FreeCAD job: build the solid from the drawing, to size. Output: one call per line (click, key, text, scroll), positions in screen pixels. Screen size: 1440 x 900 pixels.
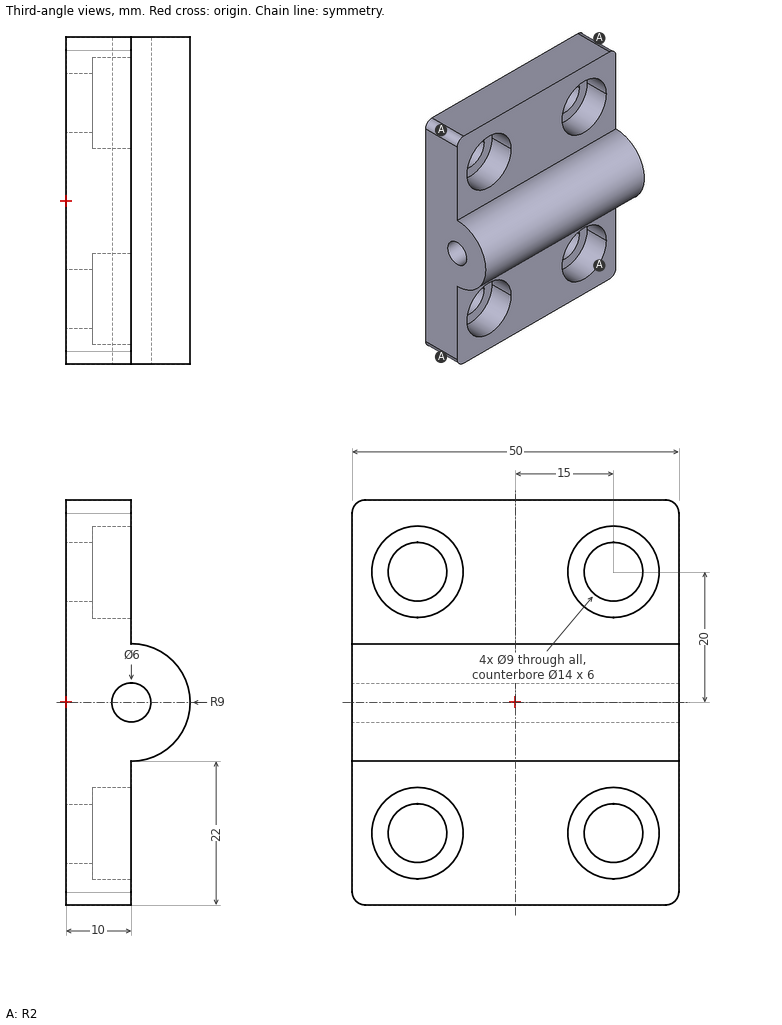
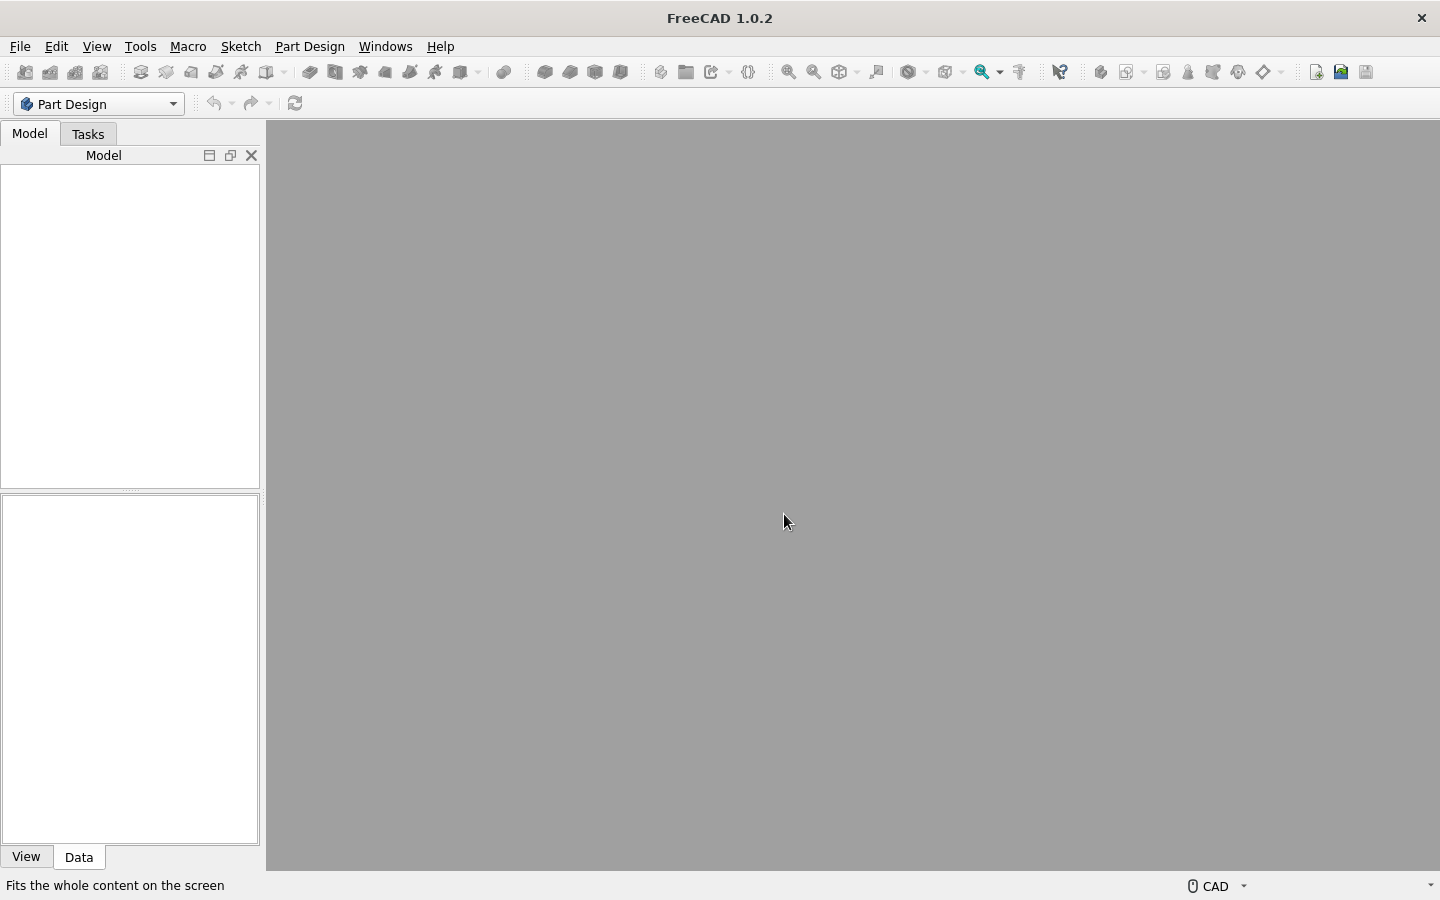
click(1316, 72)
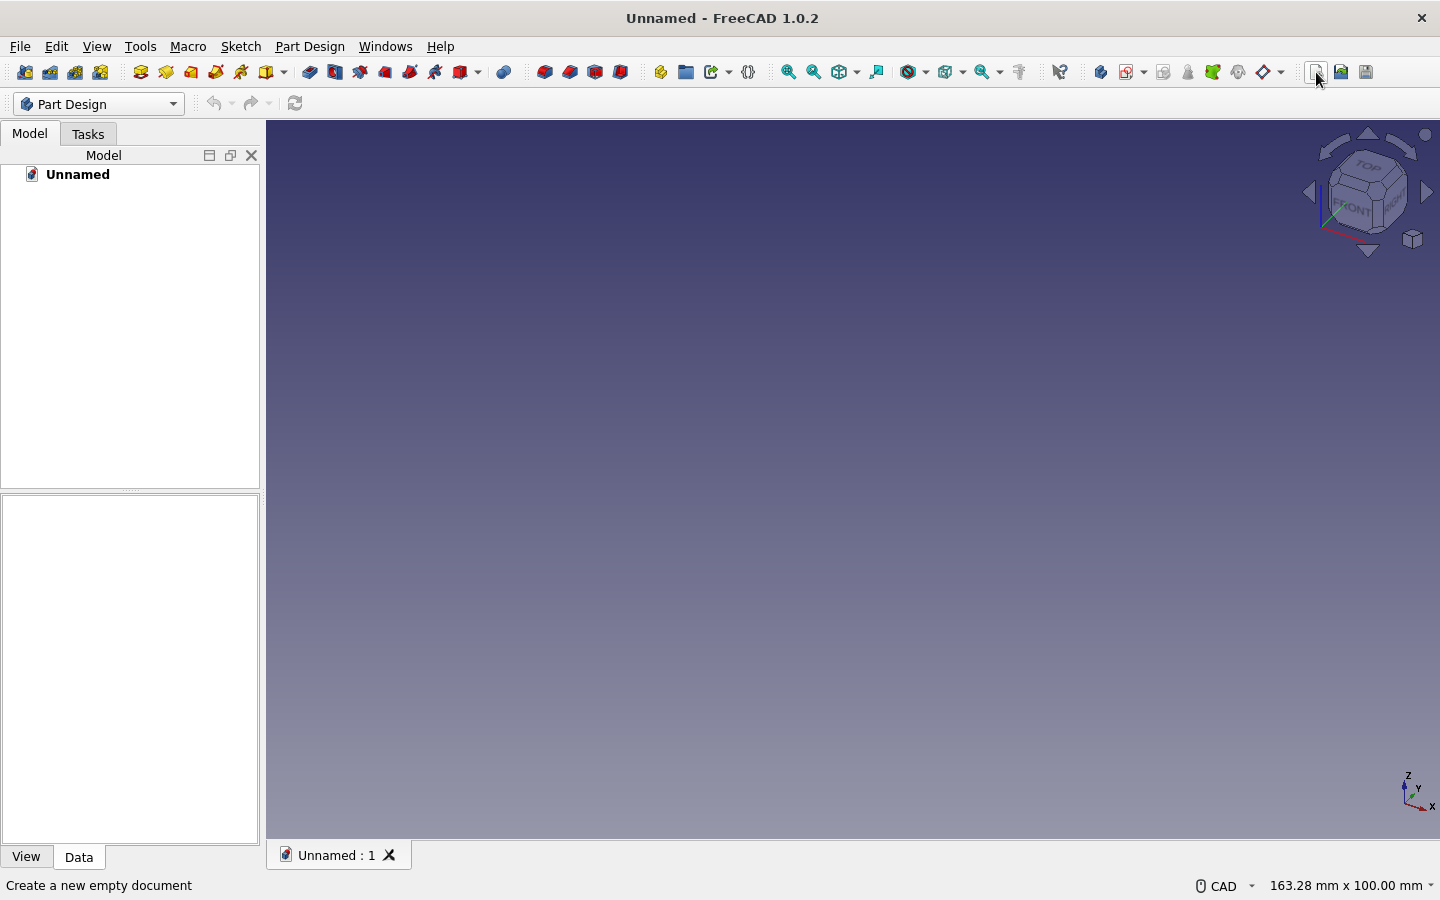
click(1126, 72)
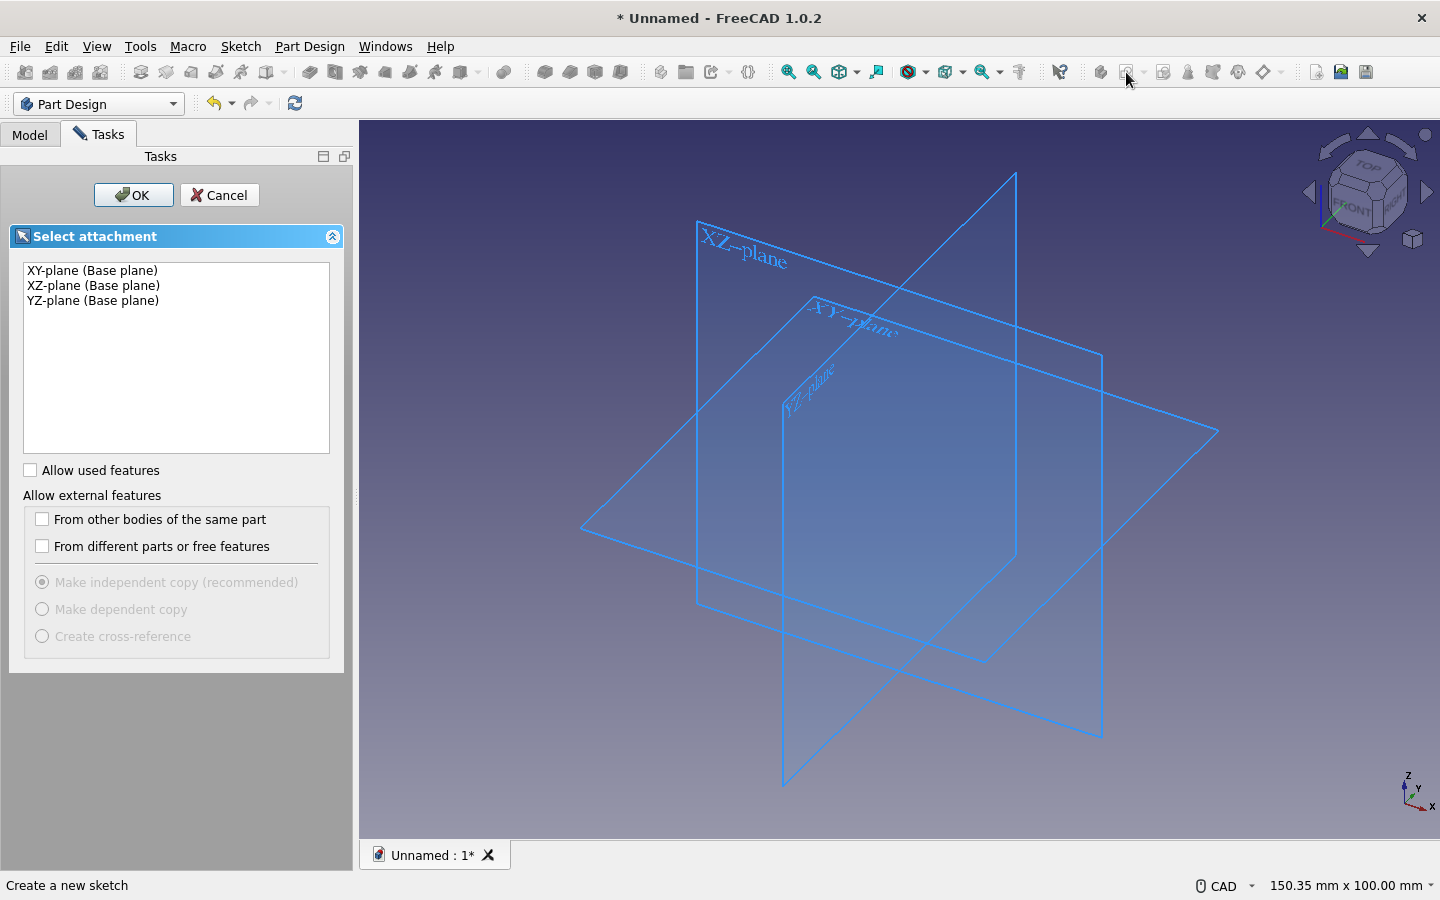
click(84, 286)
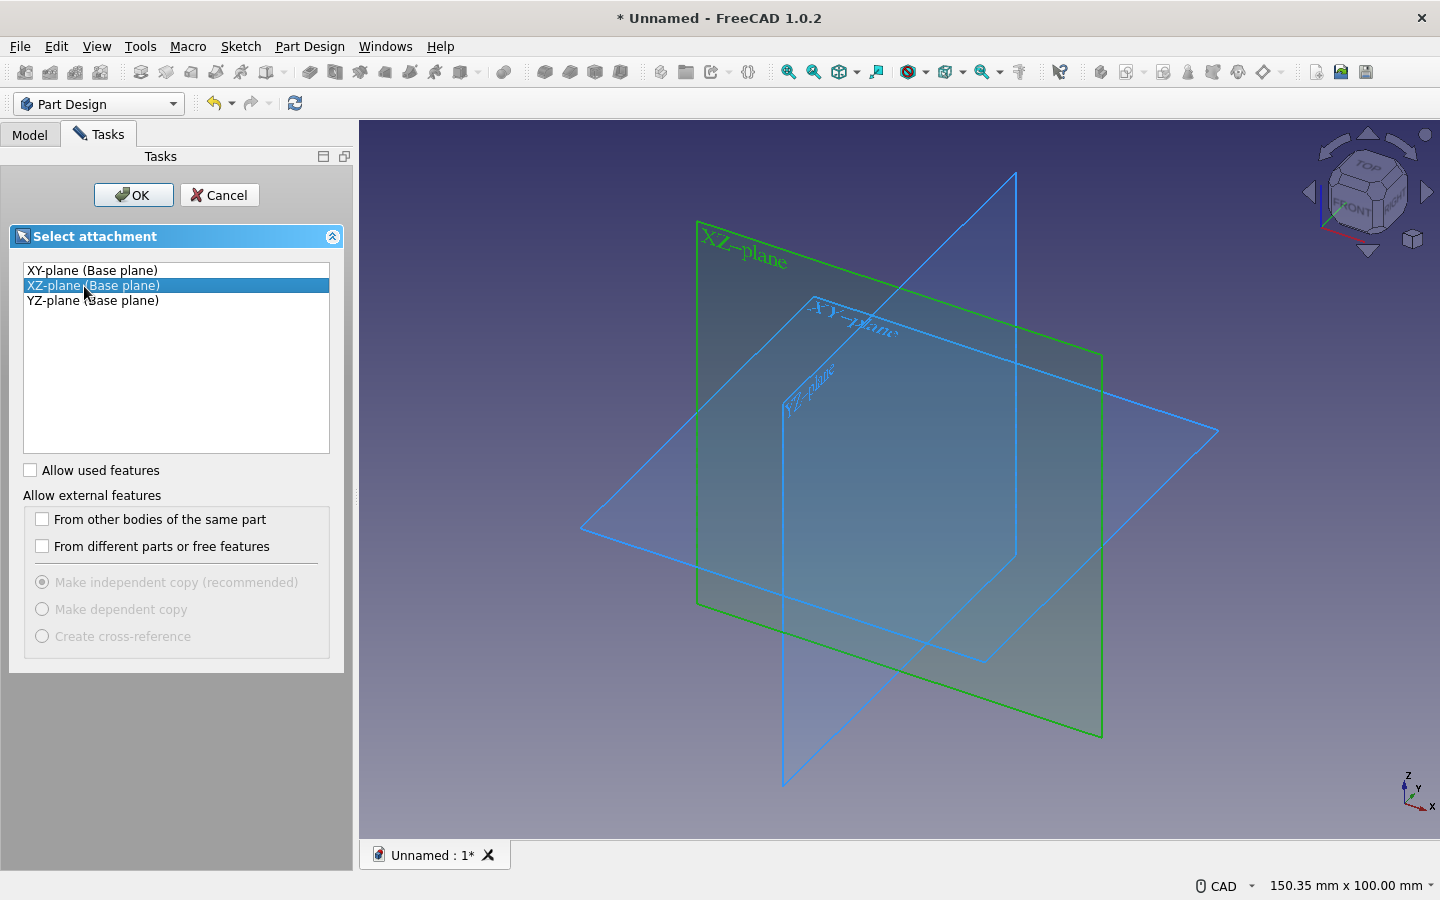
click(134, 195)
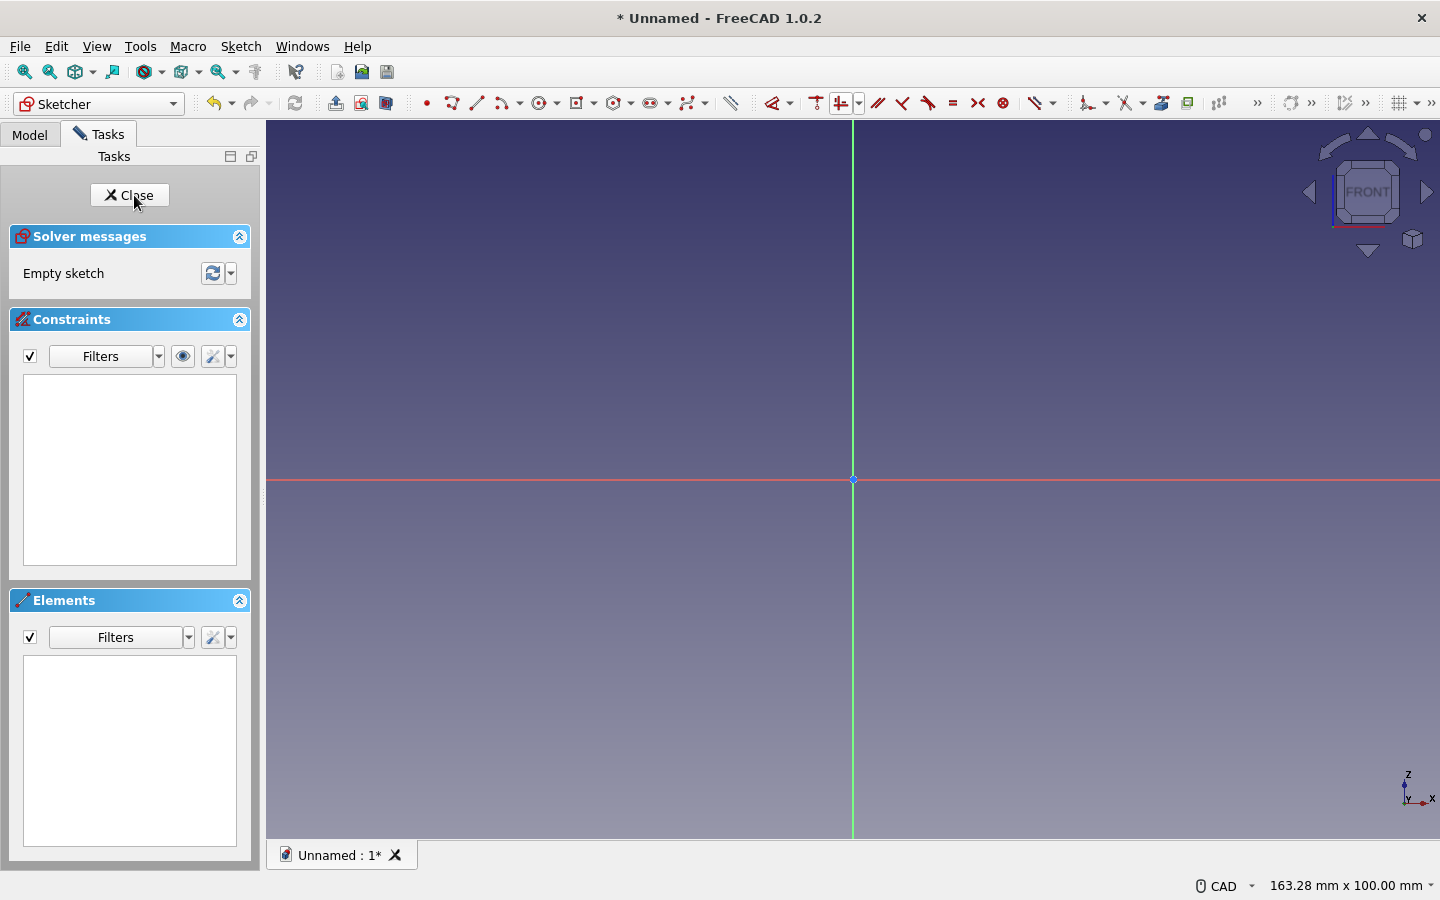
click(452, 104)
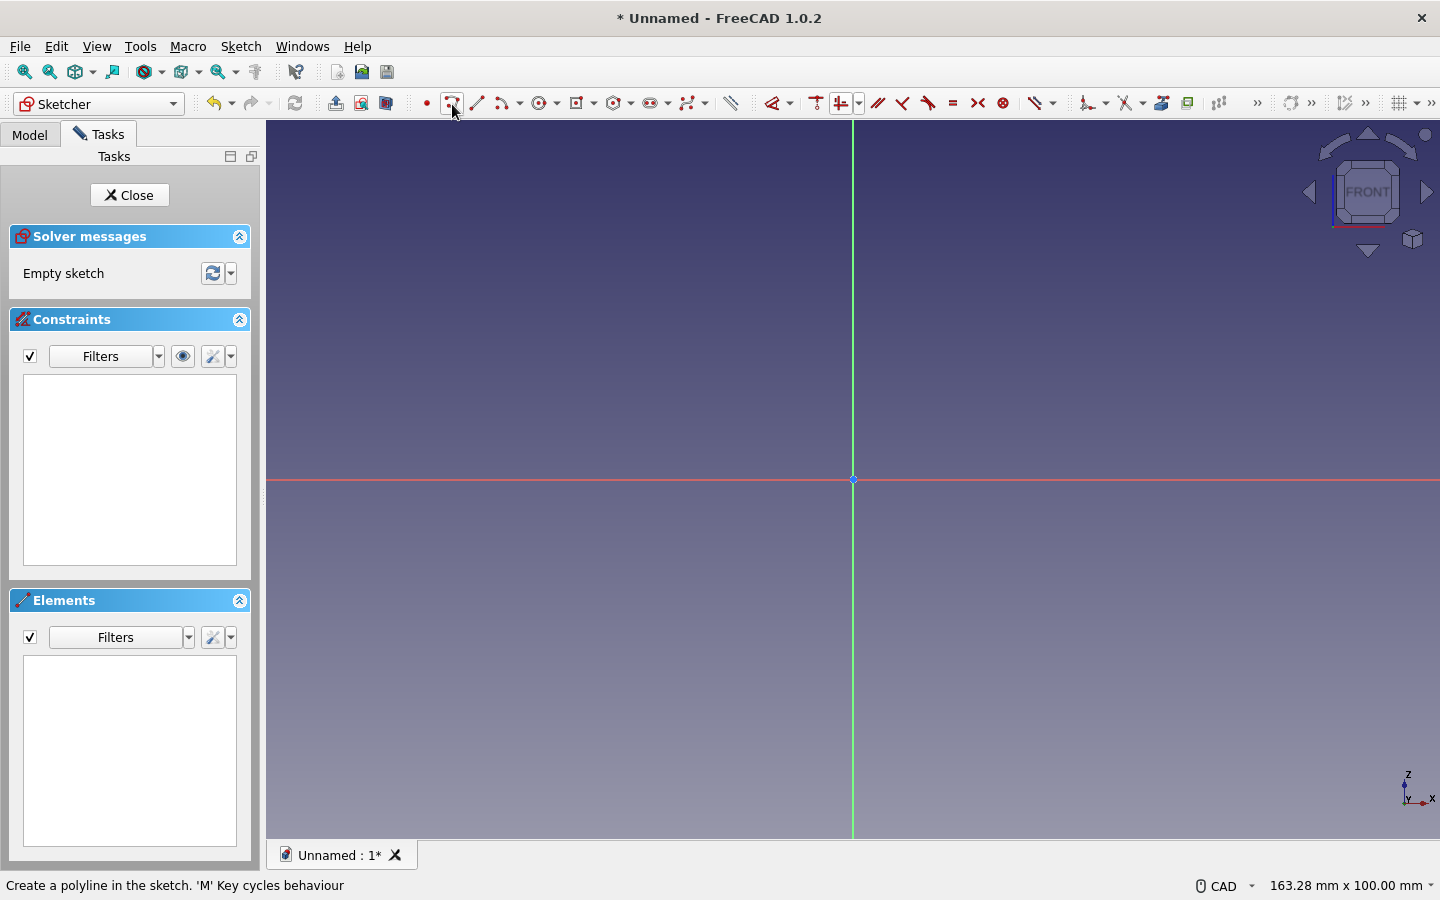
click(925, 544)
click(925, 702)
click(853, 702)
click(862, 257)
click(925, 257)
click(925, 415)
right_click(925, 415)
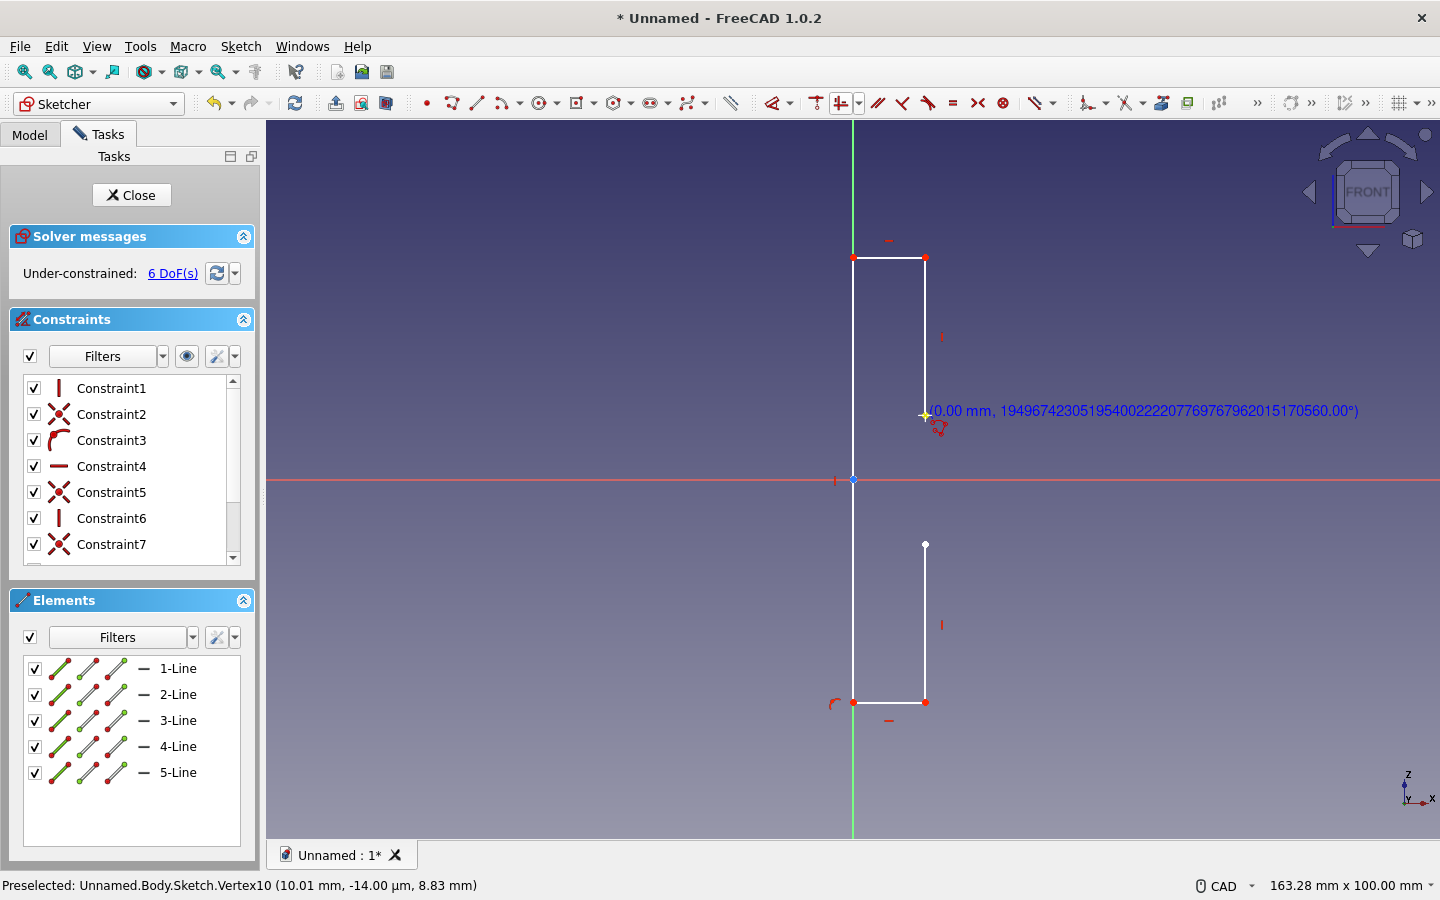
click(520, 104)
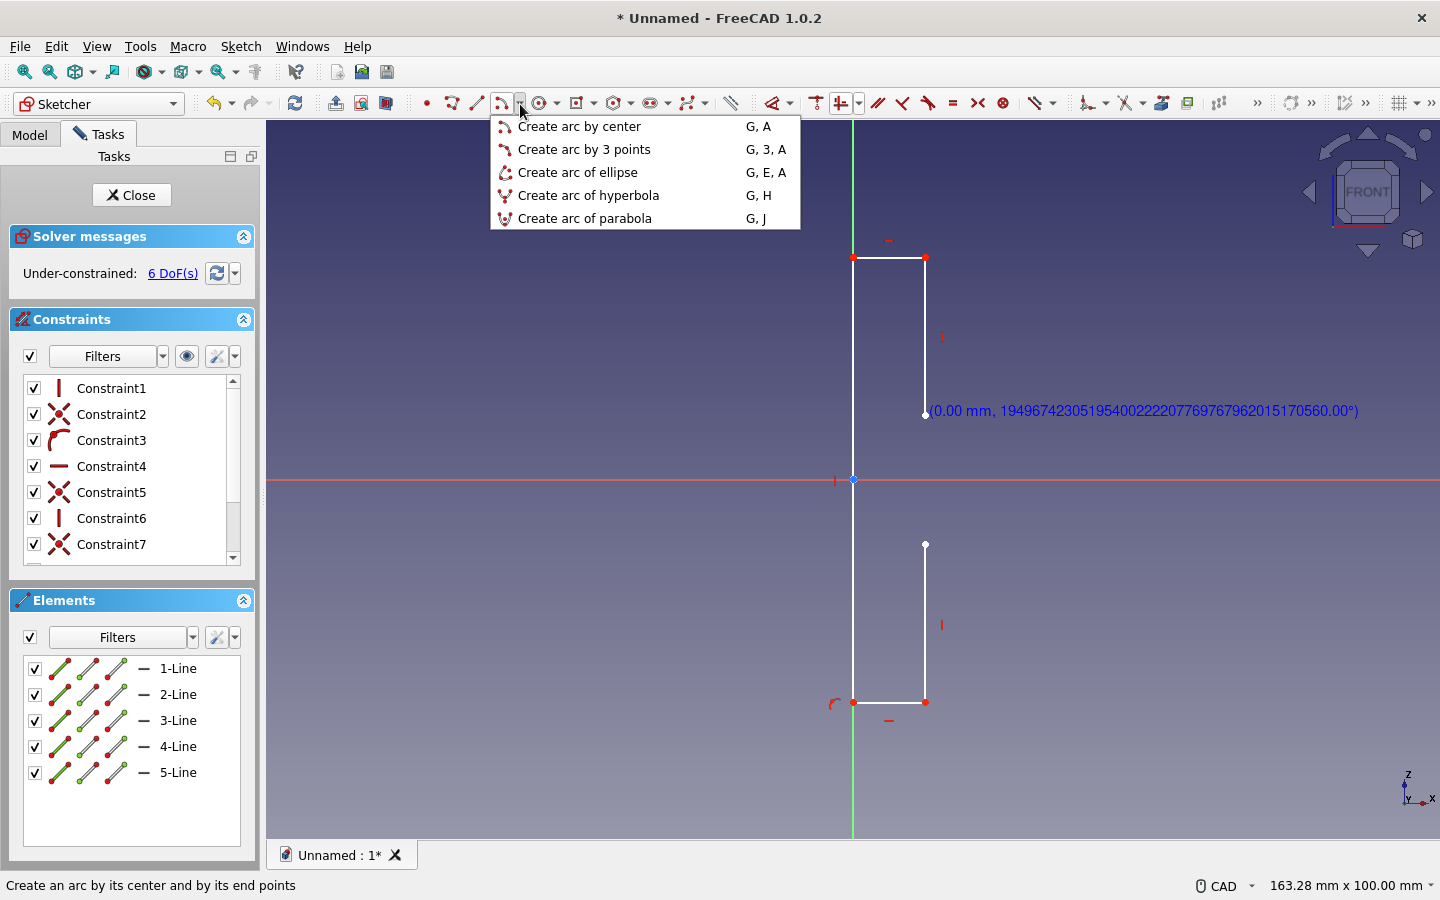
click(646, 150)